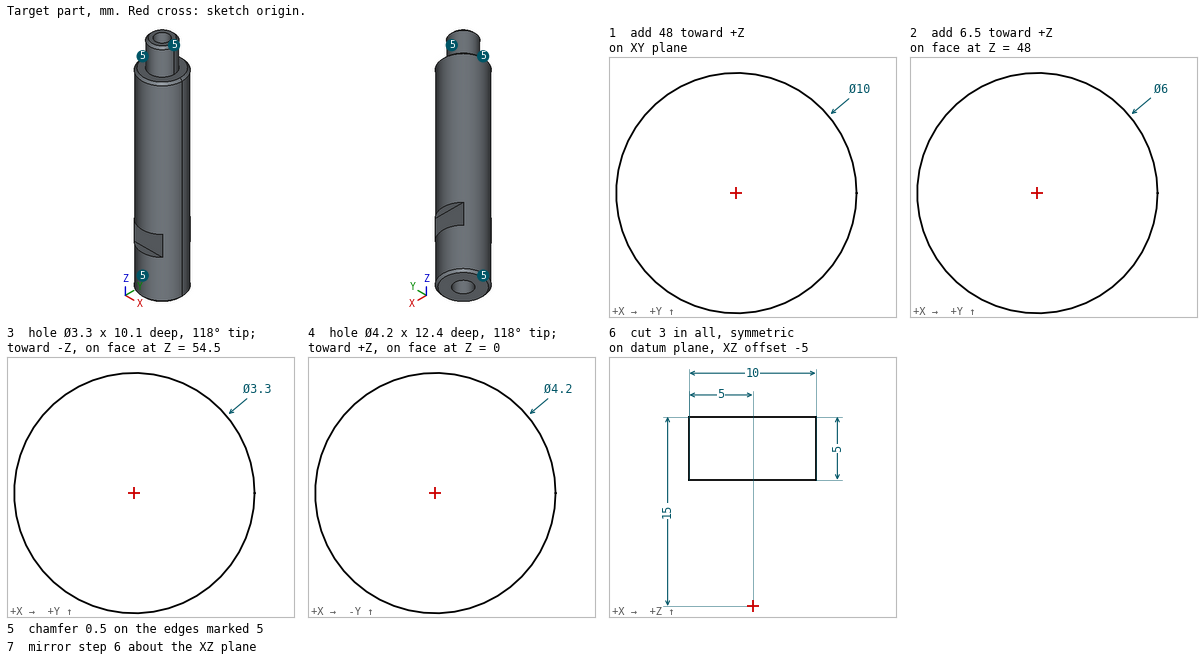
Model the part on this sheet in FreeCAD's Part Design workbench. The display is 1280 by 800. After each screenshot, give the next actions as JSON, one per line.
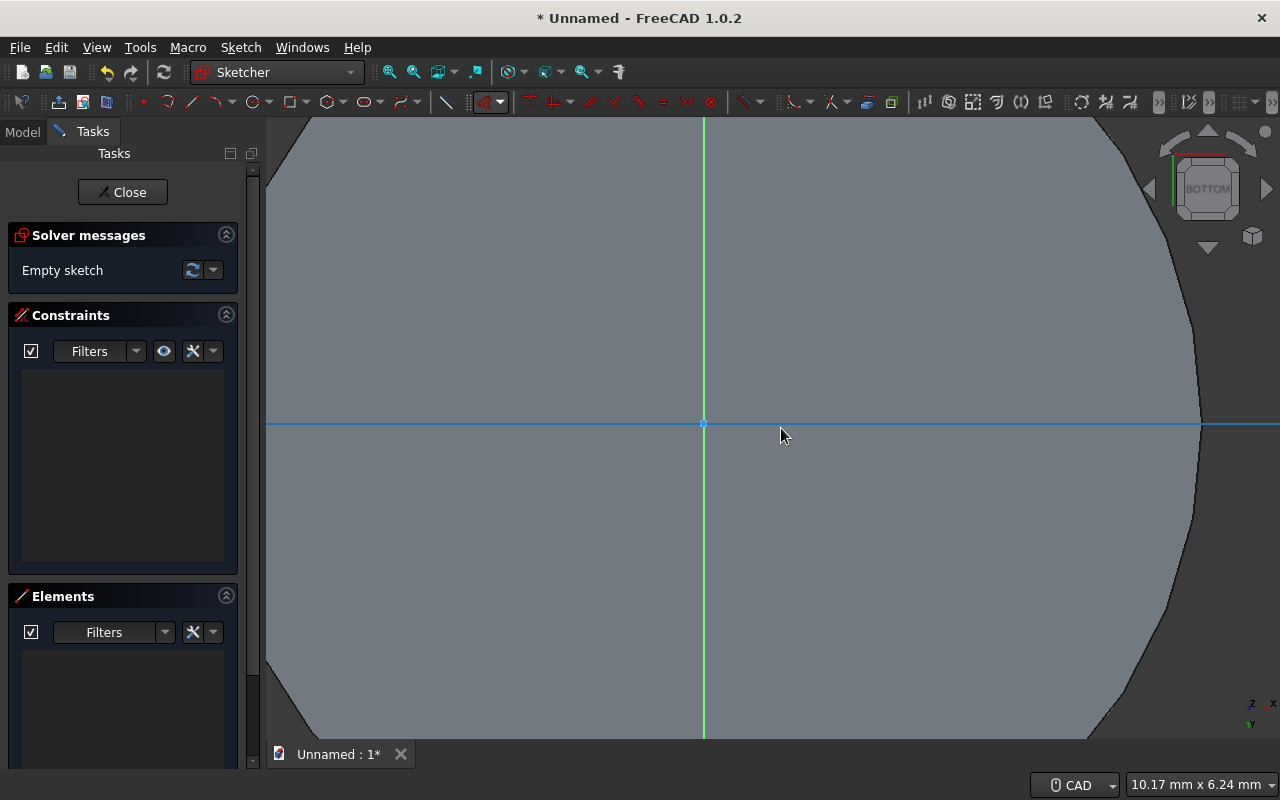
{"action": "left_click", "coordinate": [254, 102]}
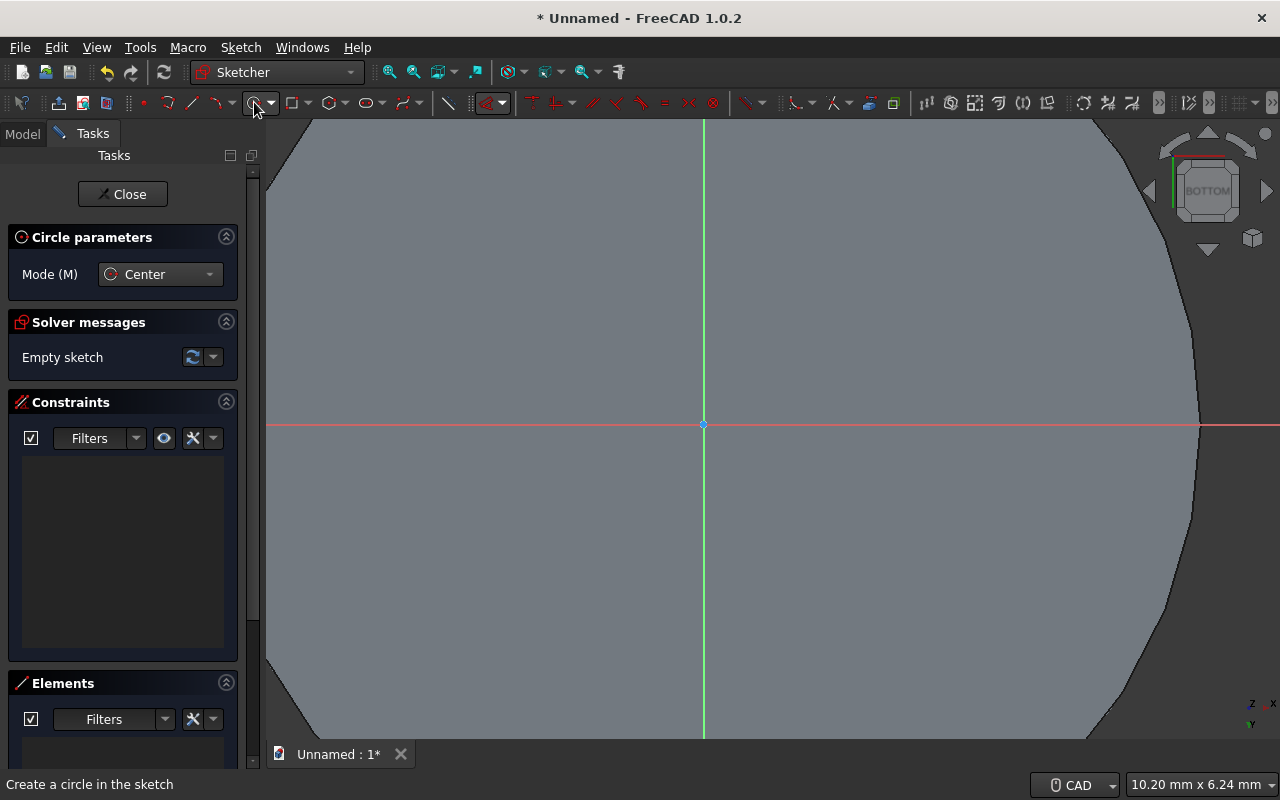
{"action": "left_click", "coordinate": [704, 425]}
{"action": "mouse_move", "coordinate": [851, 277]}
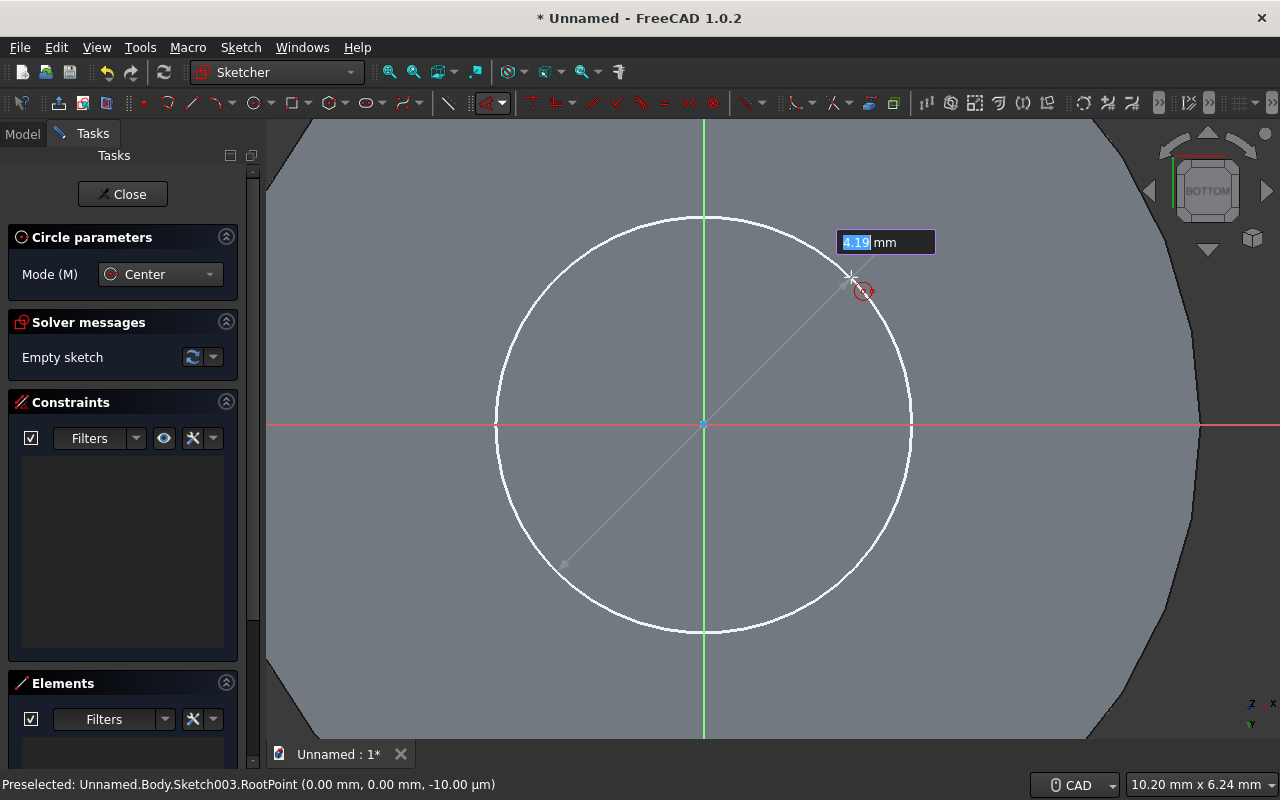
{"action": "type", "text": "4.2"}
{"action": "key", "text": "Return"}
{"action": "key", "text": "Escape"}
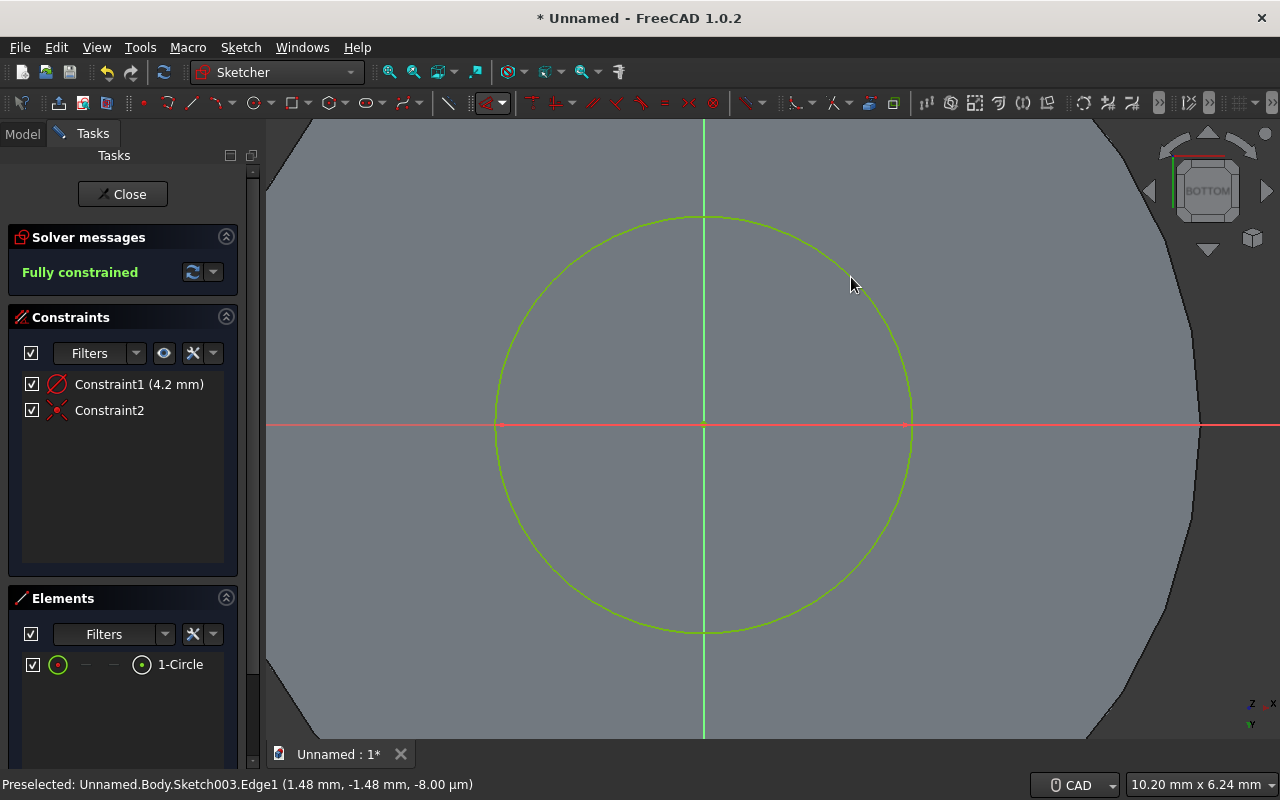
{"action": "left_click", "coordinate": [123, 194]}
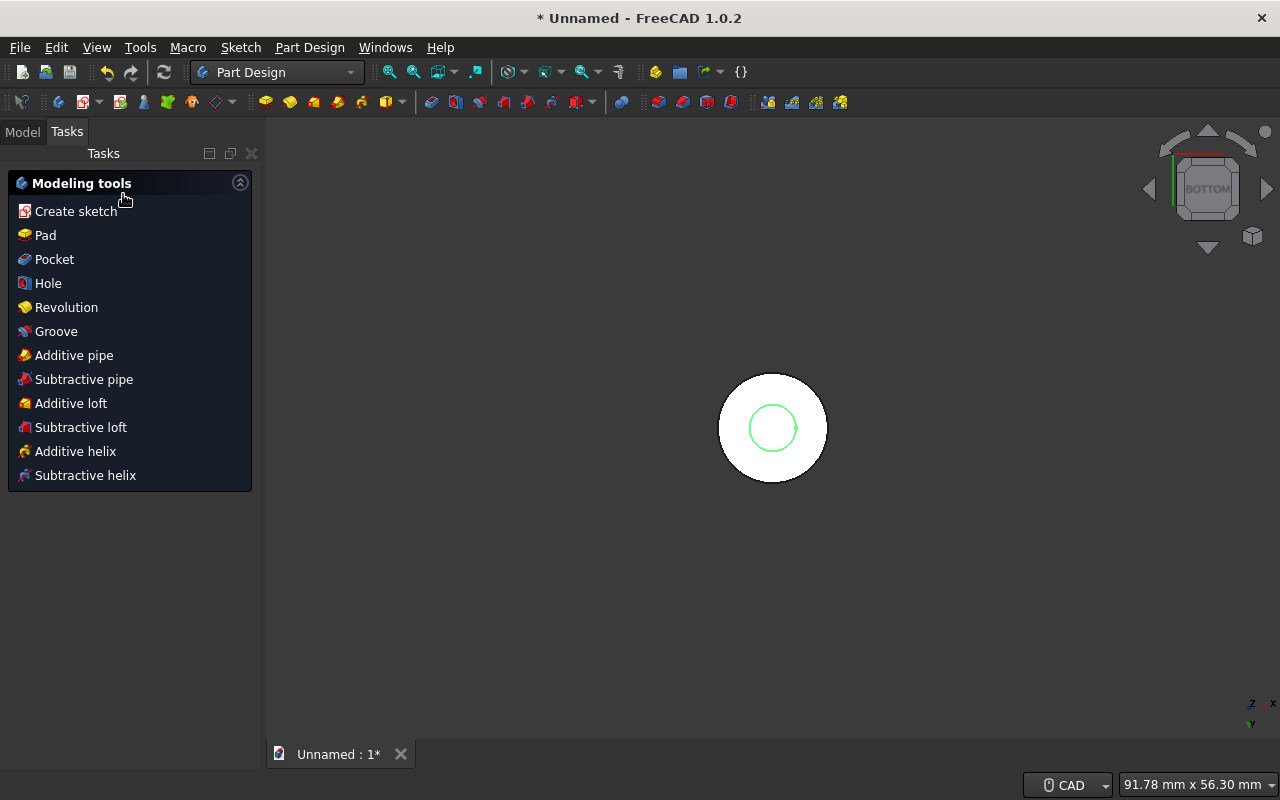
{"action": "left_click", "coordinate": [456, 102]}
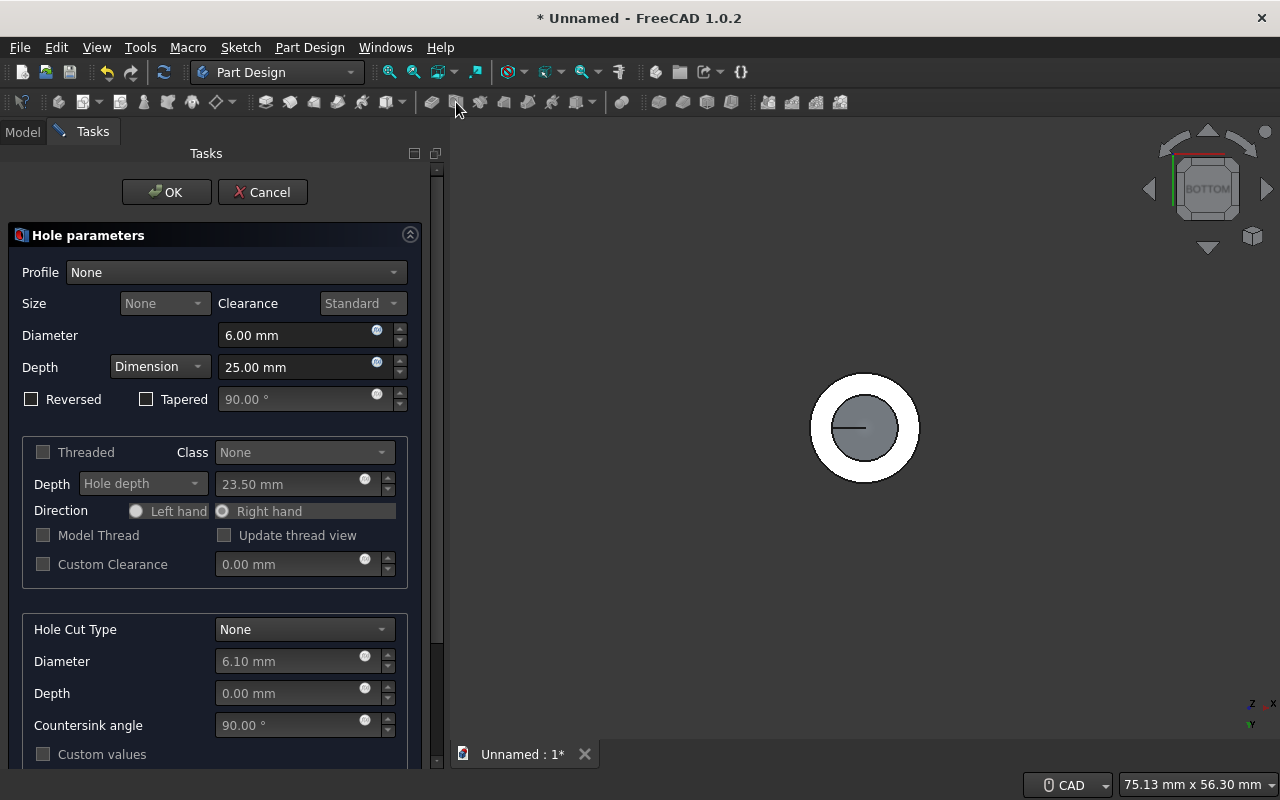
{"action": "triple_click", "coordinate": [305, 335]}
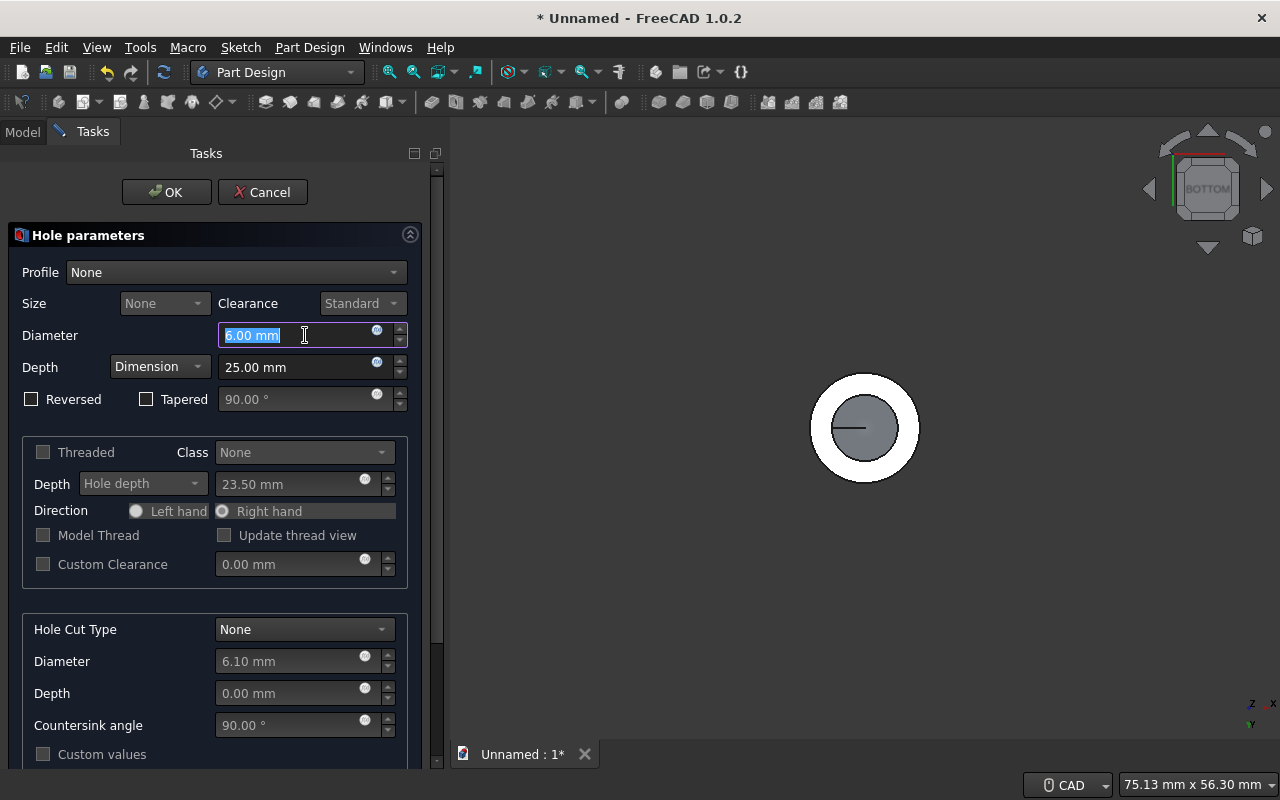
{"action": "type", "text": "4.2"}
{"action": "key", "text": "Tab"}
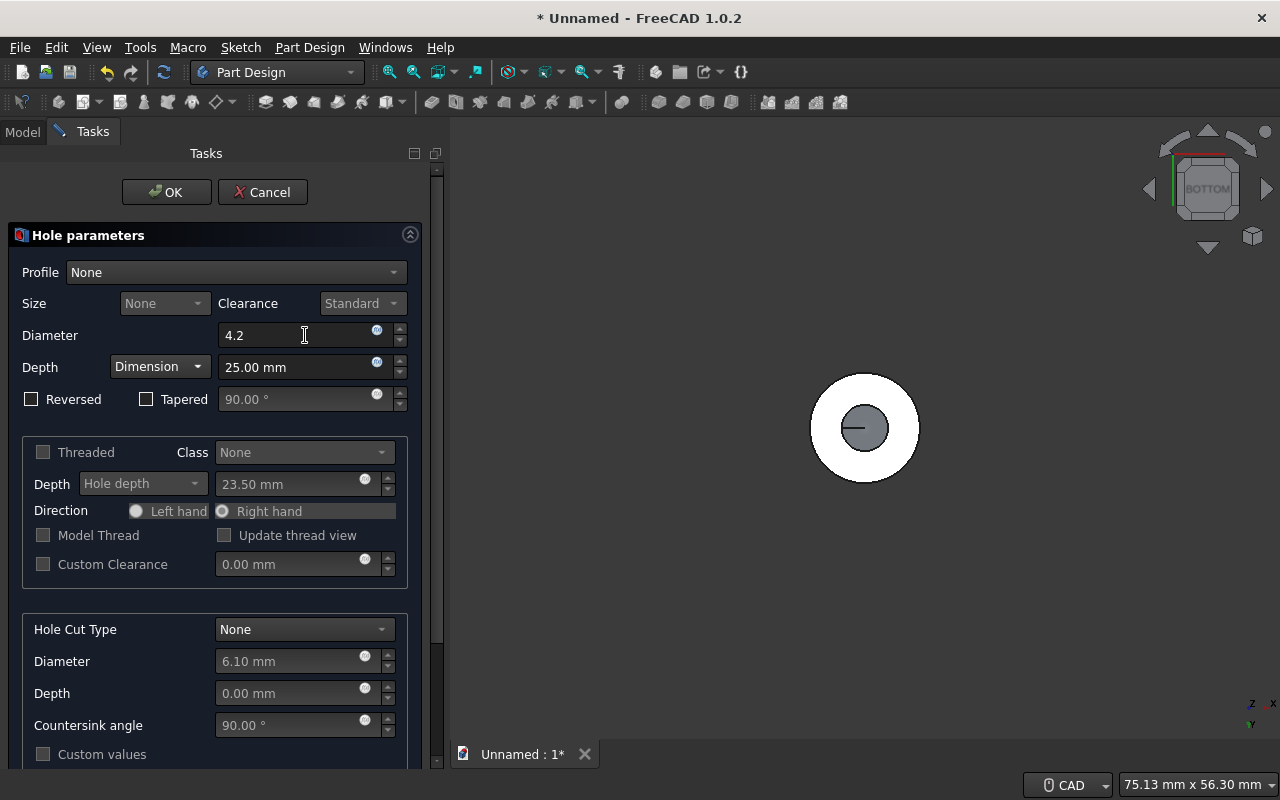
{"action": "triple_click", "coordinate": [305, 367]}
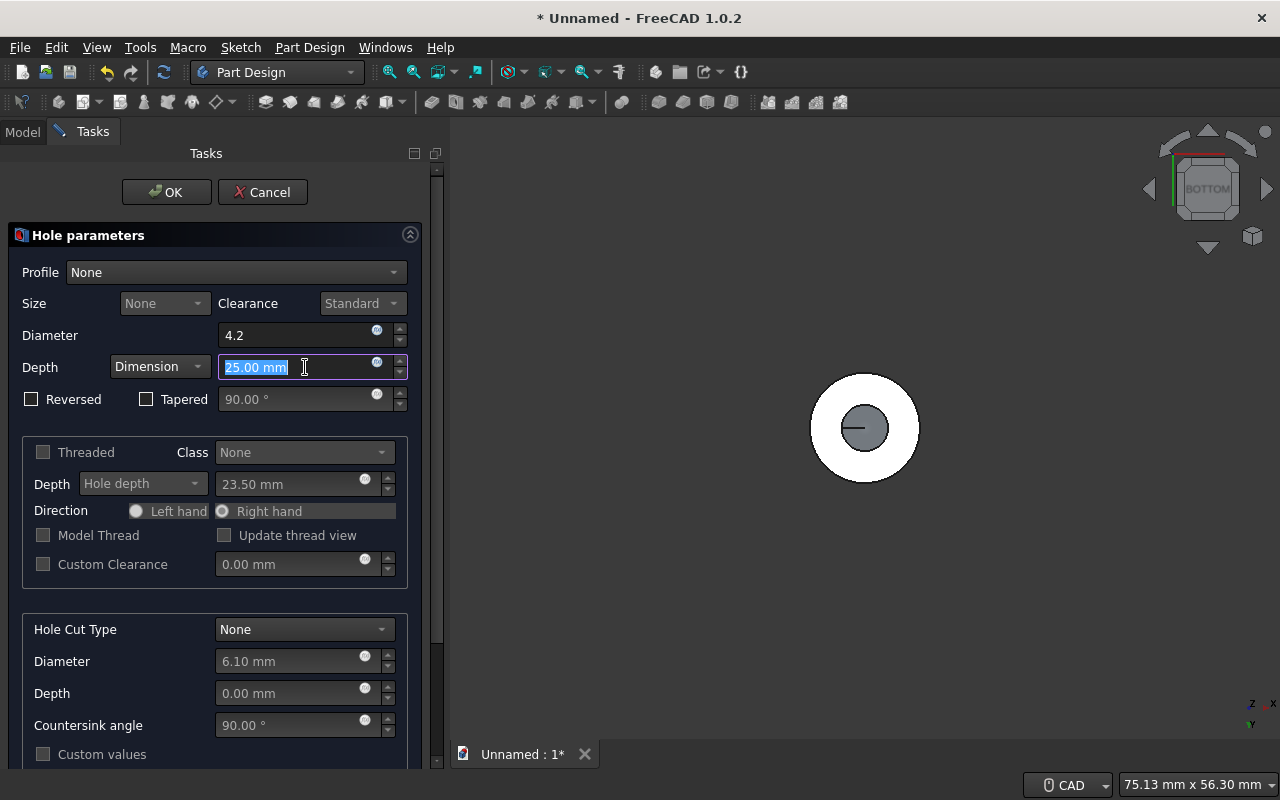
{"action": "type", "text": "12.4"}
{"action": "key", "text": "Tab"}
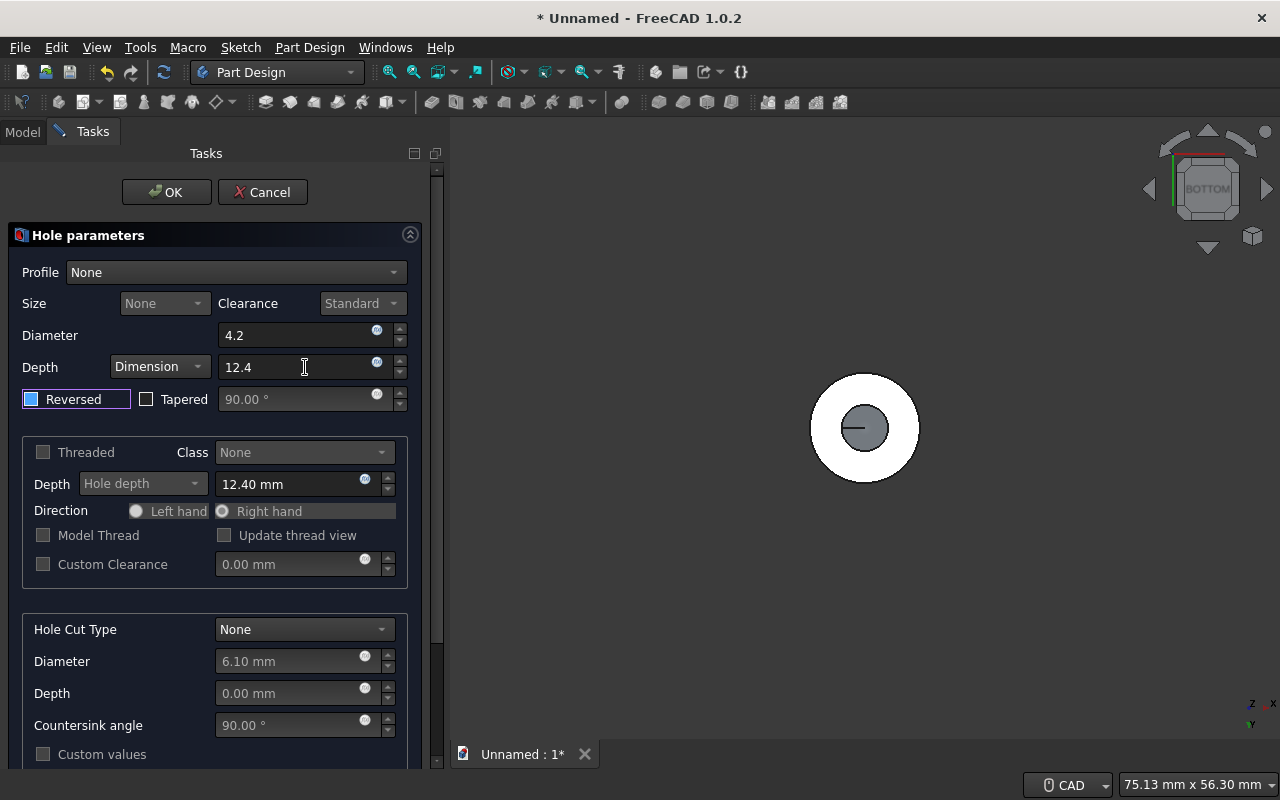
{"action": "left_click", "coordinate": [167, 192]}